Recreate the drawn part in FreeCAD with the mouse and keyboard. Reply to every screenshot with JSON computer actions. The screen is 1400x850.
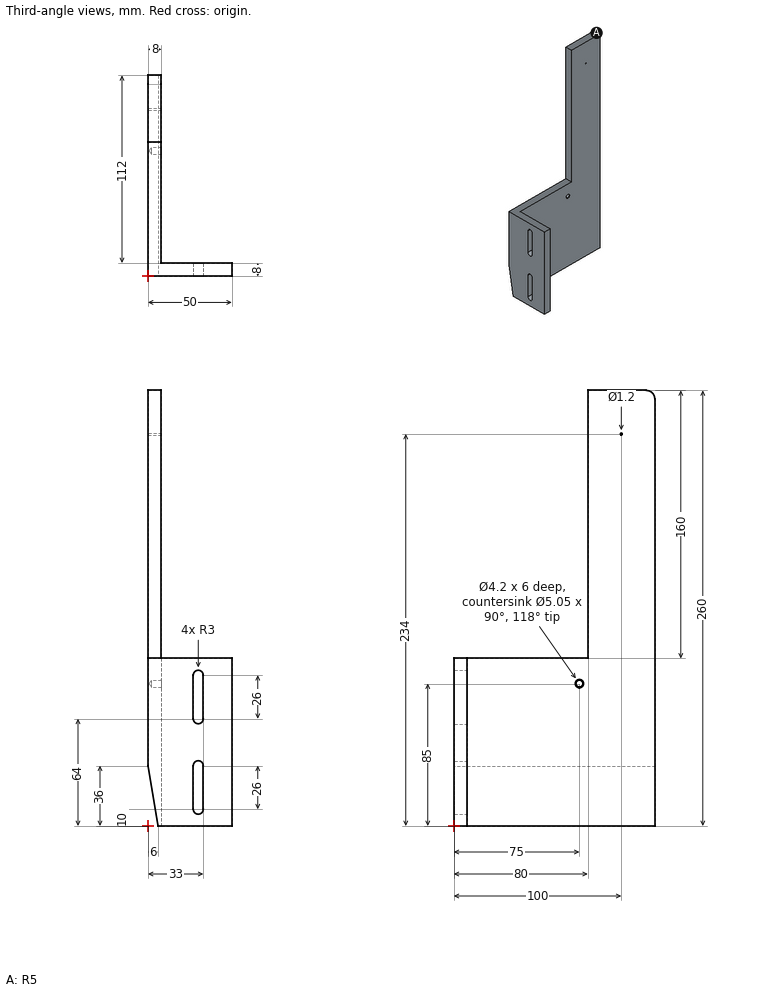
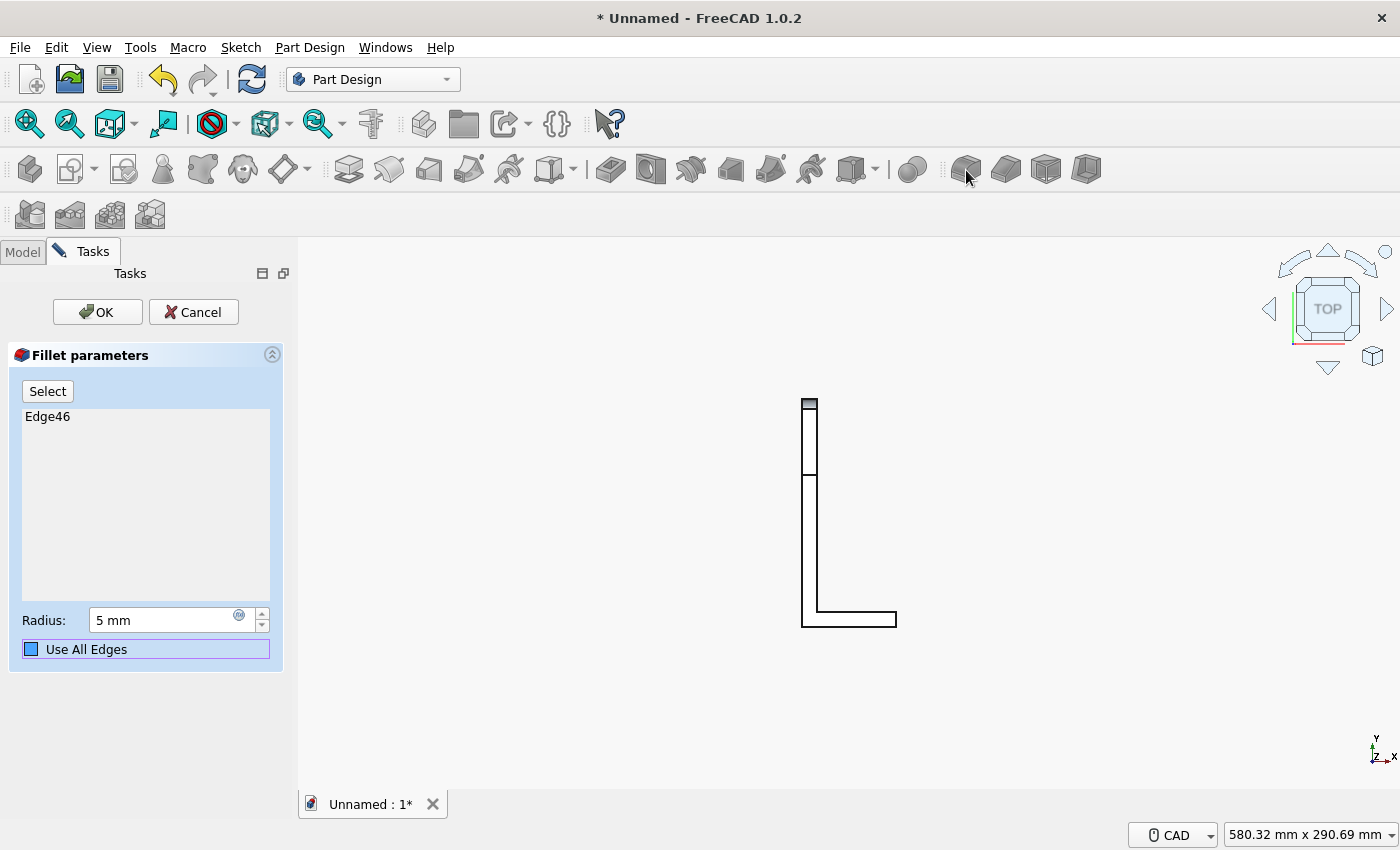
{"action": "left_click", "coordinate": [98, 312]}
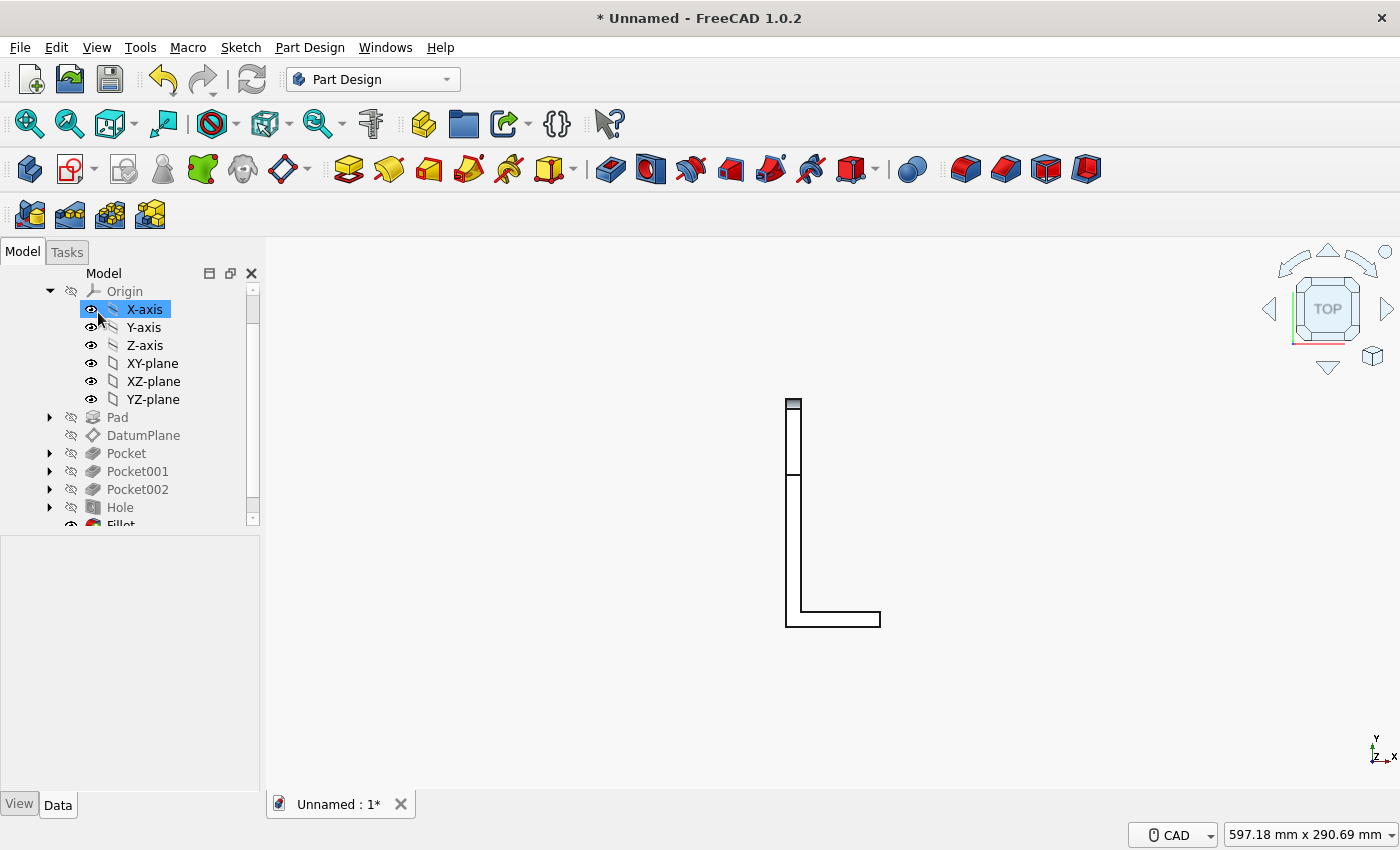
{"action": "left_click", "coordinate": [30, 124]}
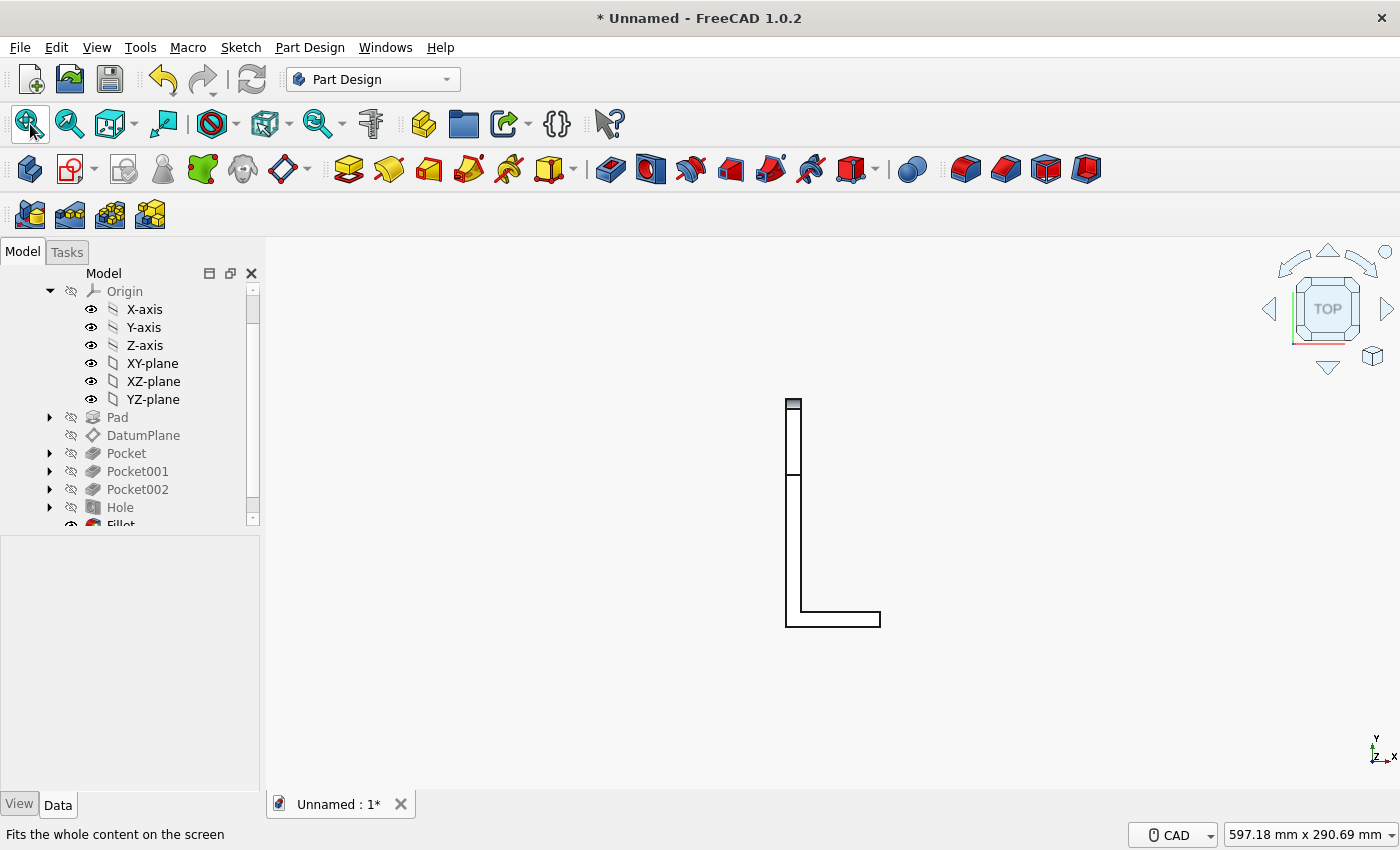
{"action": "key", "text": "0"}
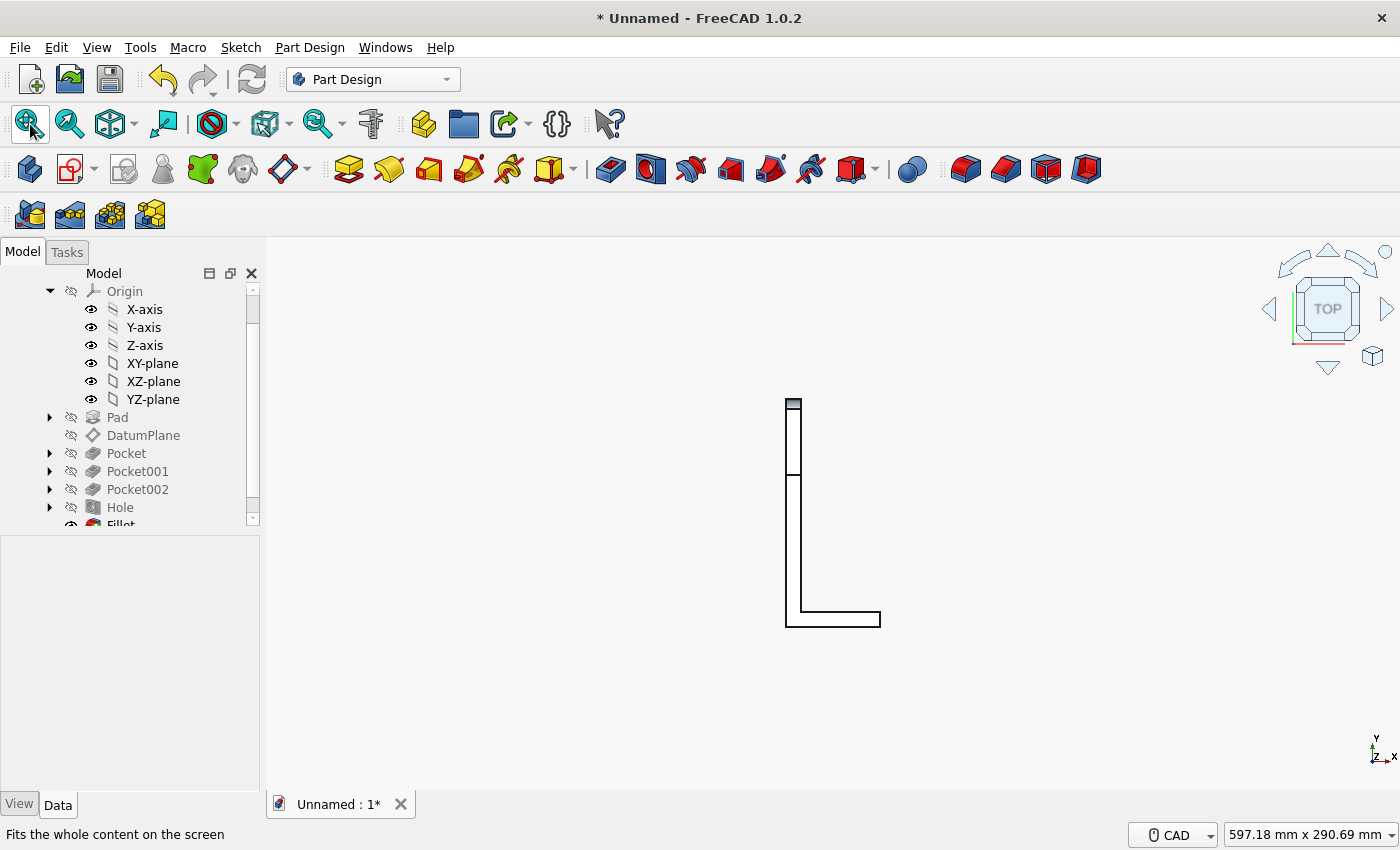
{"action": "left_click", "coordinate": [816, 611]}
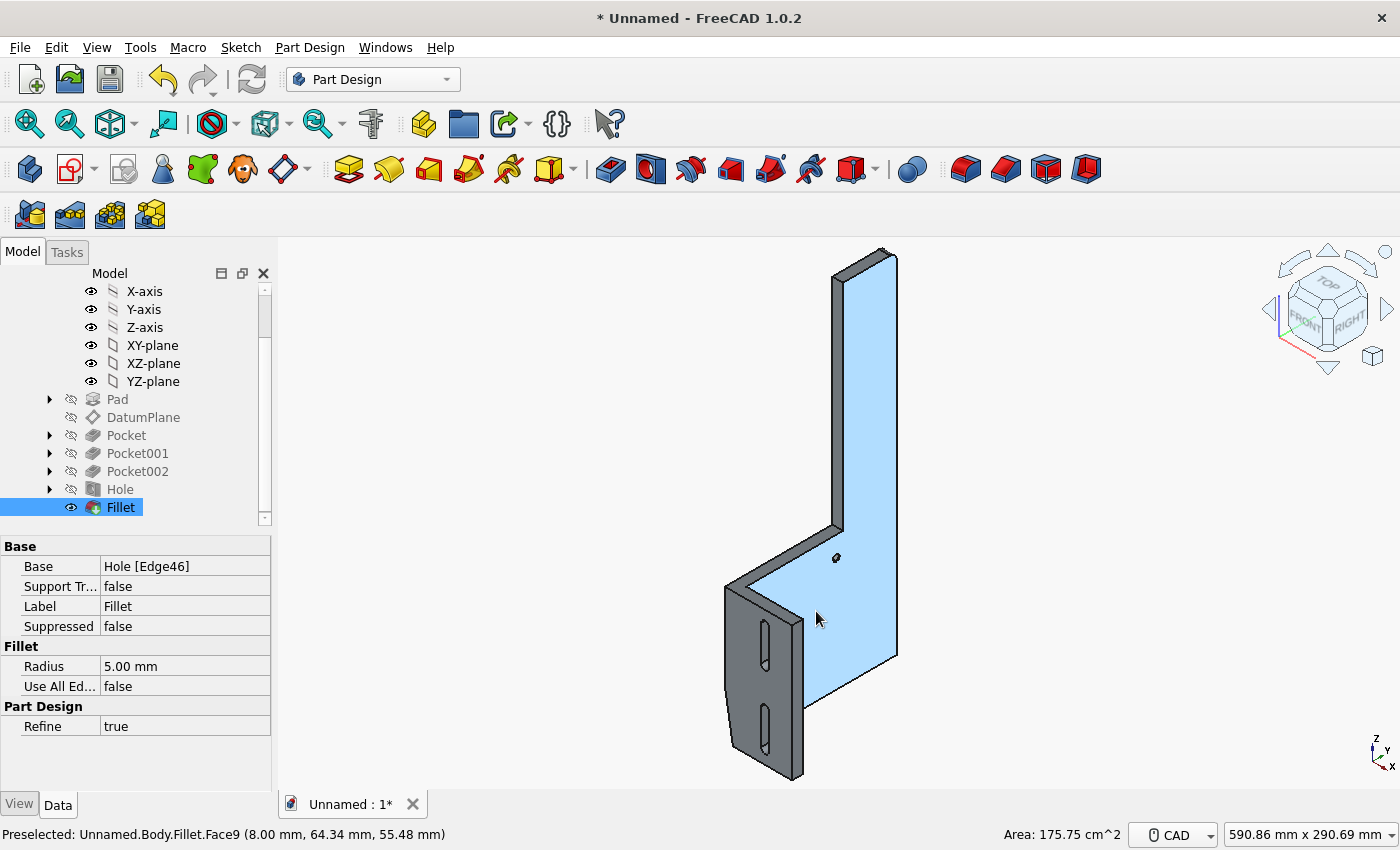
{"action": "left_click", "coordinate": [70, 170]}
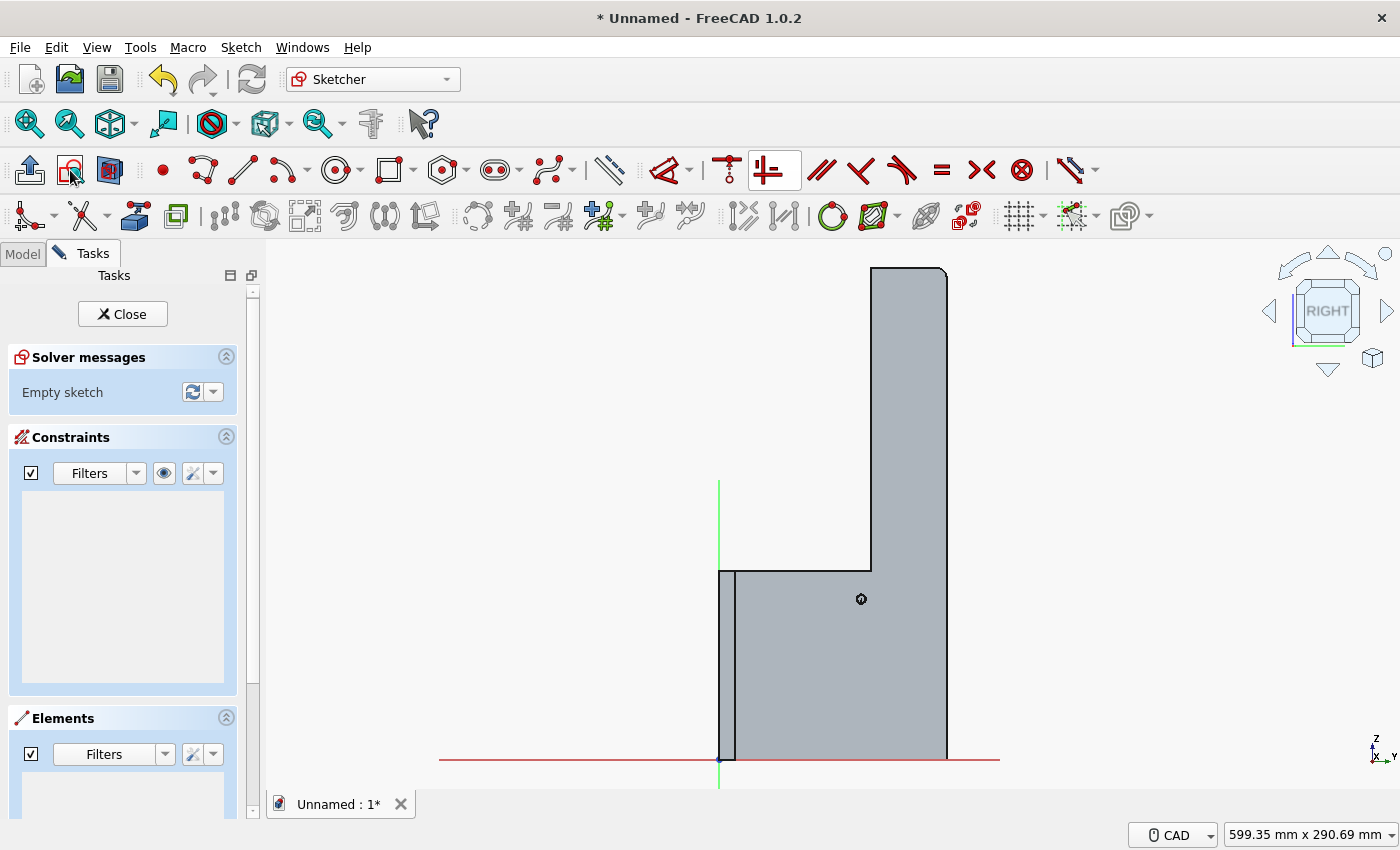
{"action": "scroll", "coordinate": [916, 307], "scroll_direction": "up", "scroll_amount": 15}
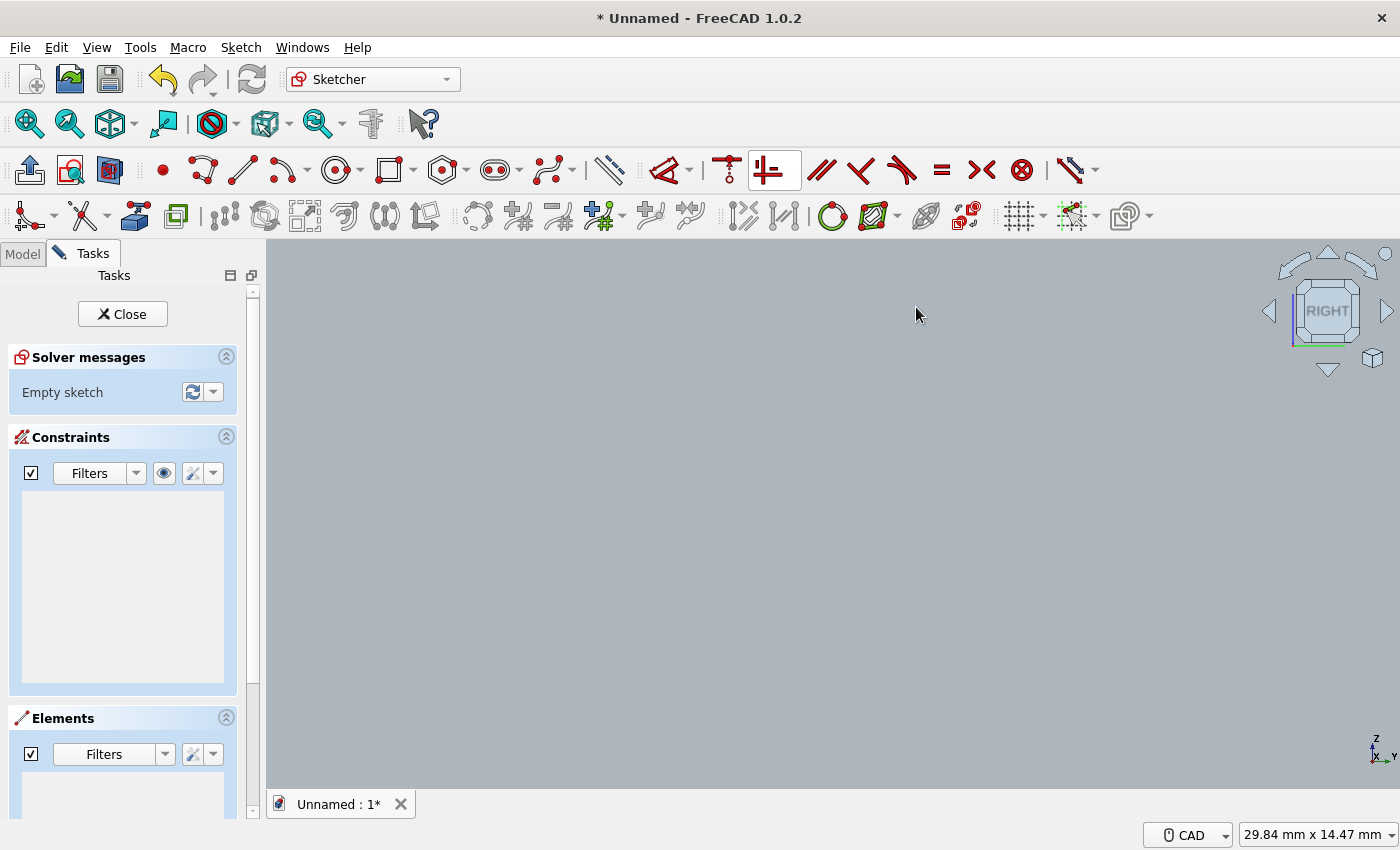
{"action": "scroll", "coordinate": [757, 509], "scroll_direction": "up", "scroll_amount": 10}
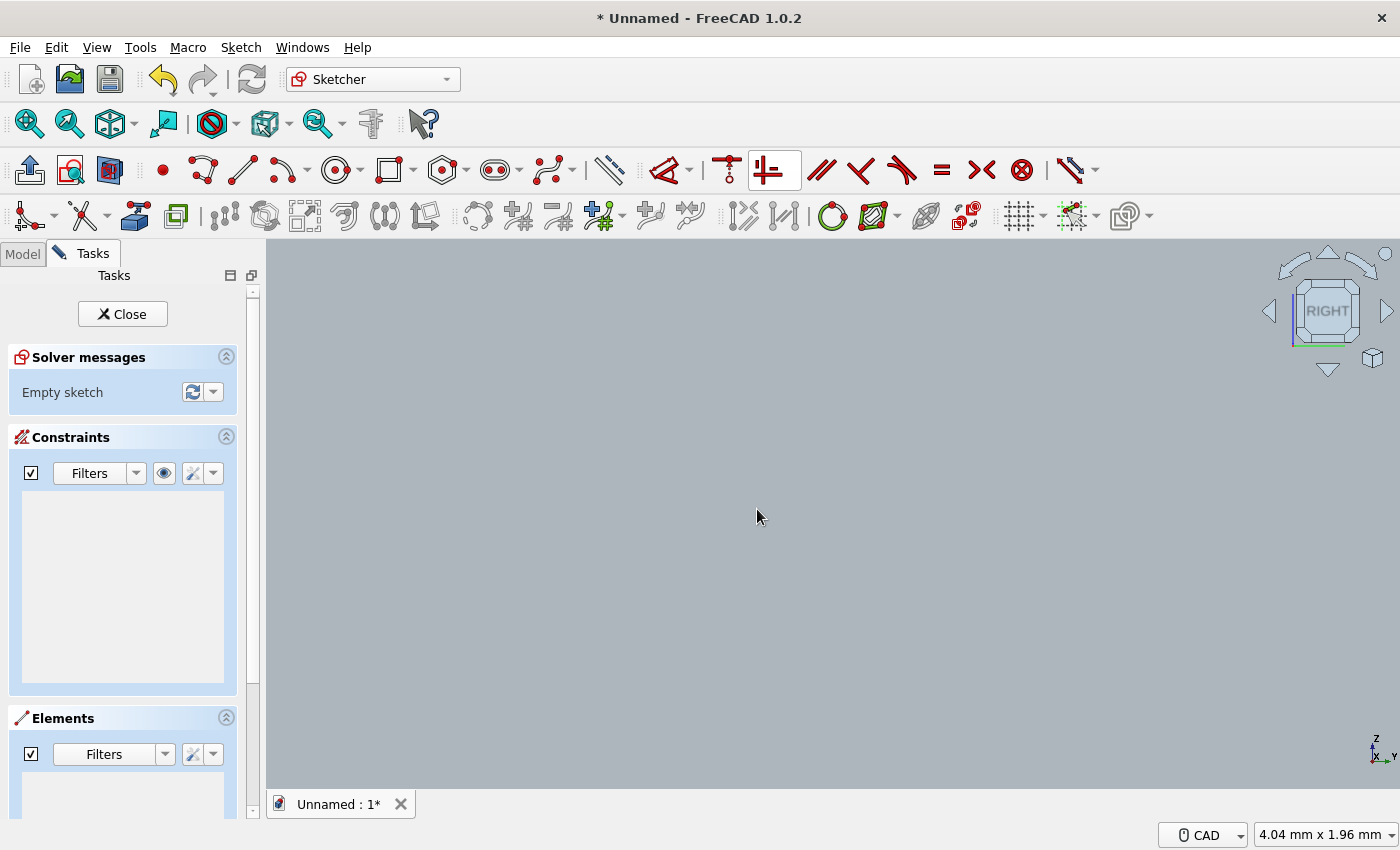
{"action": "left_click", "coordinate": [336, 170]}